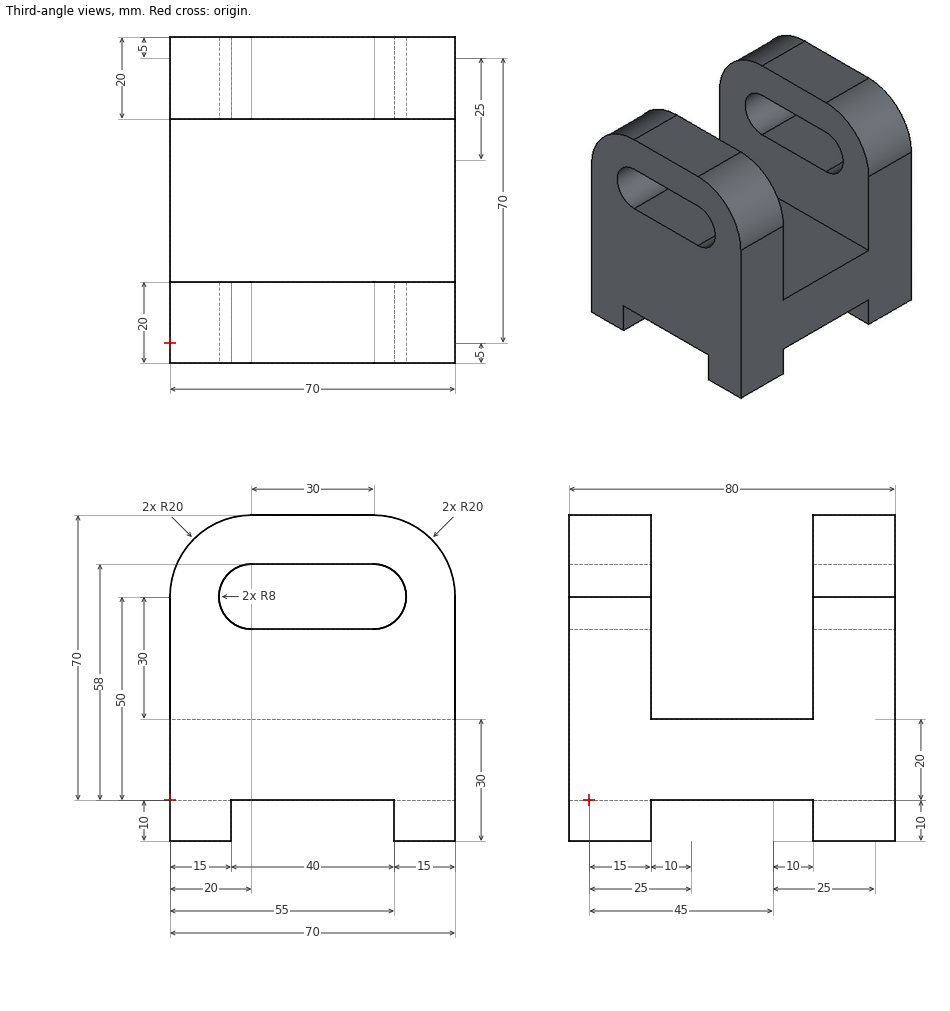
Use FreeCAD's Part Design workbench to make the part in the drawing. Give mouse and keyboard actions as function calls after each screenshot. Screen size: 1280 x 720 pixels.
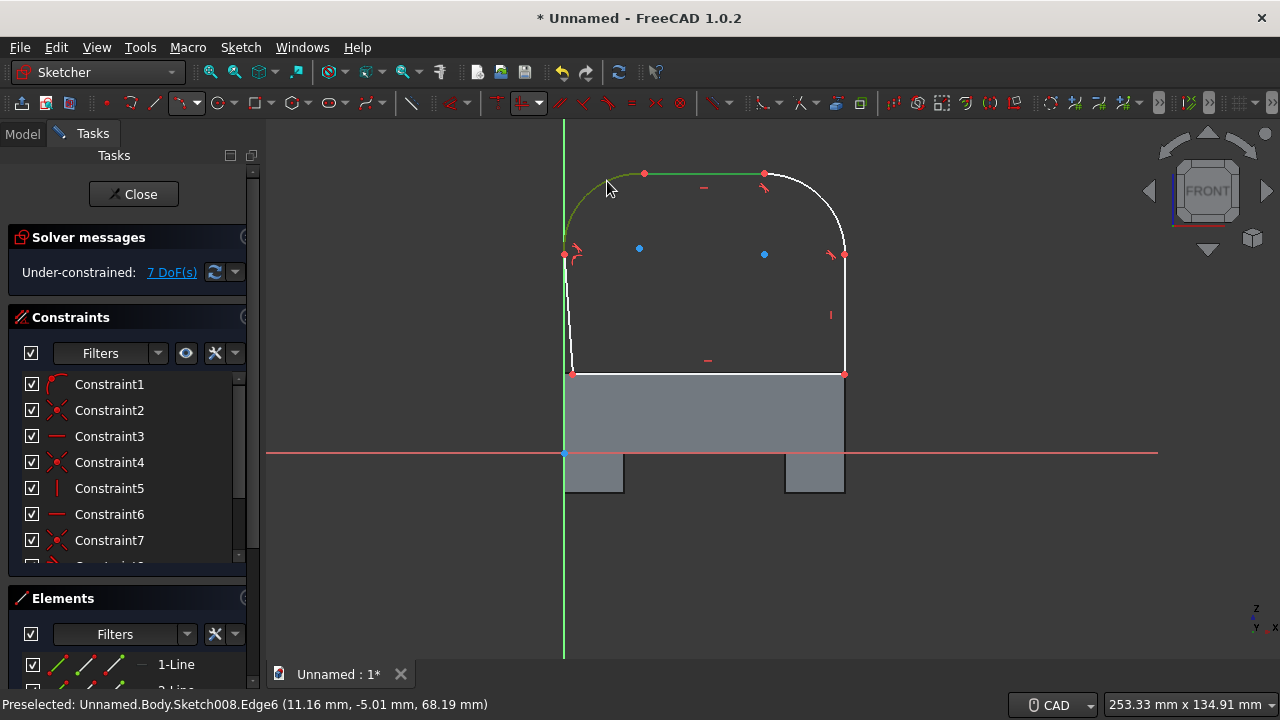
key(t)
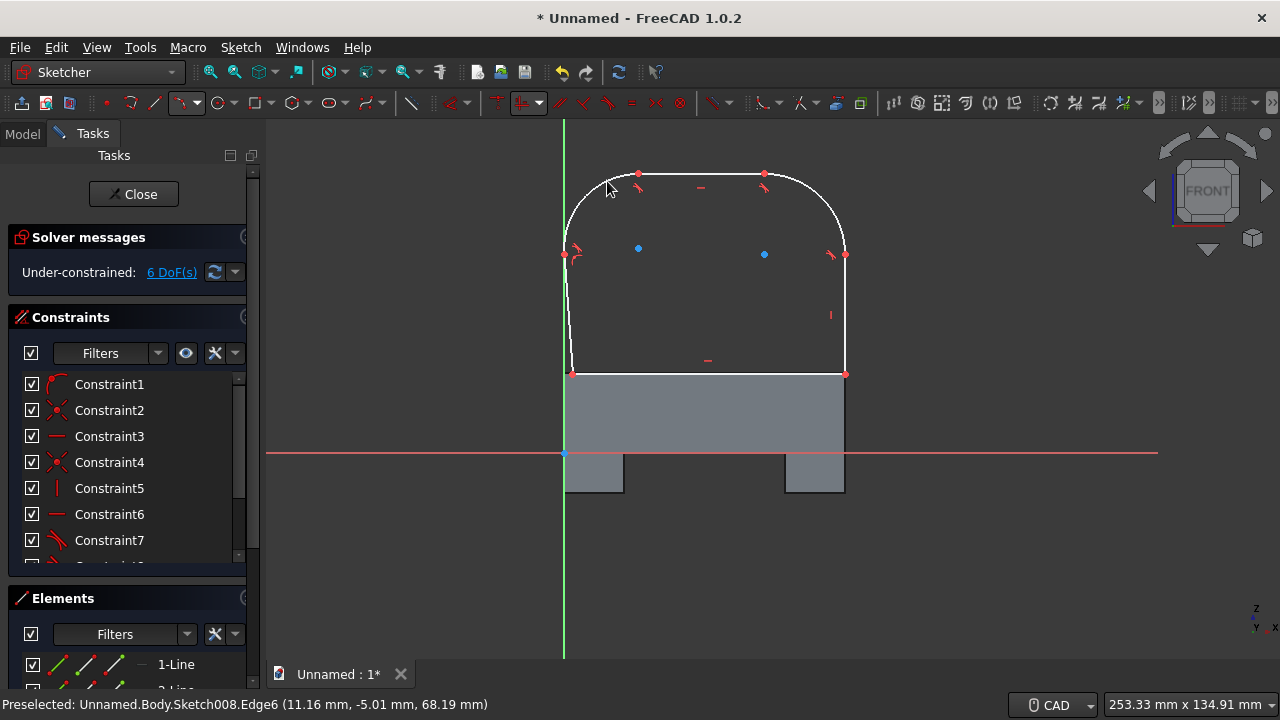
click(567, 290)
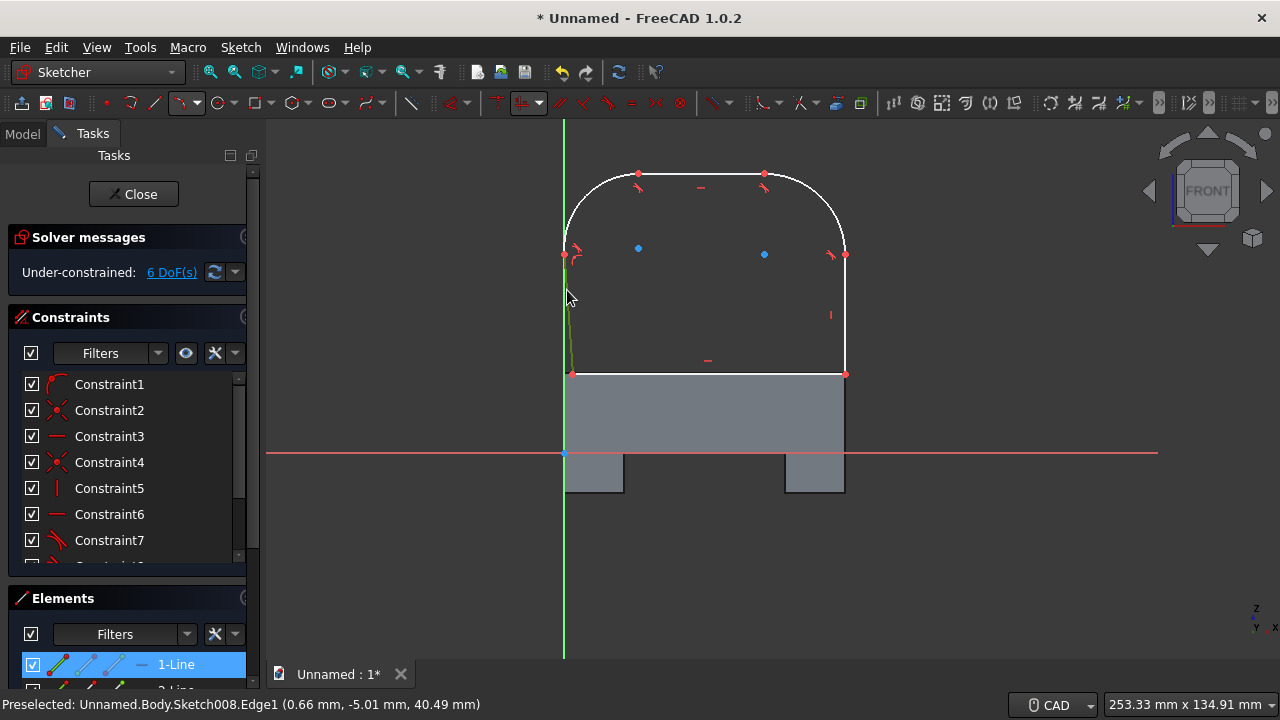
key(v)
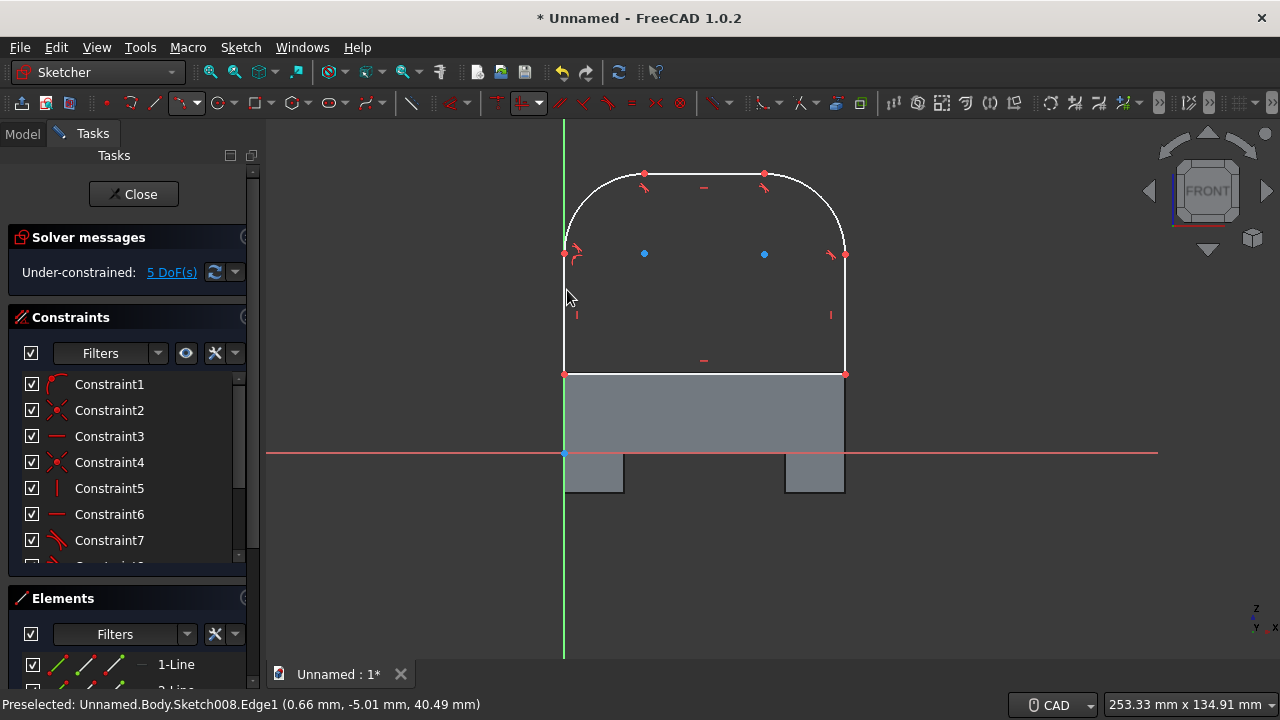
click(836, 218)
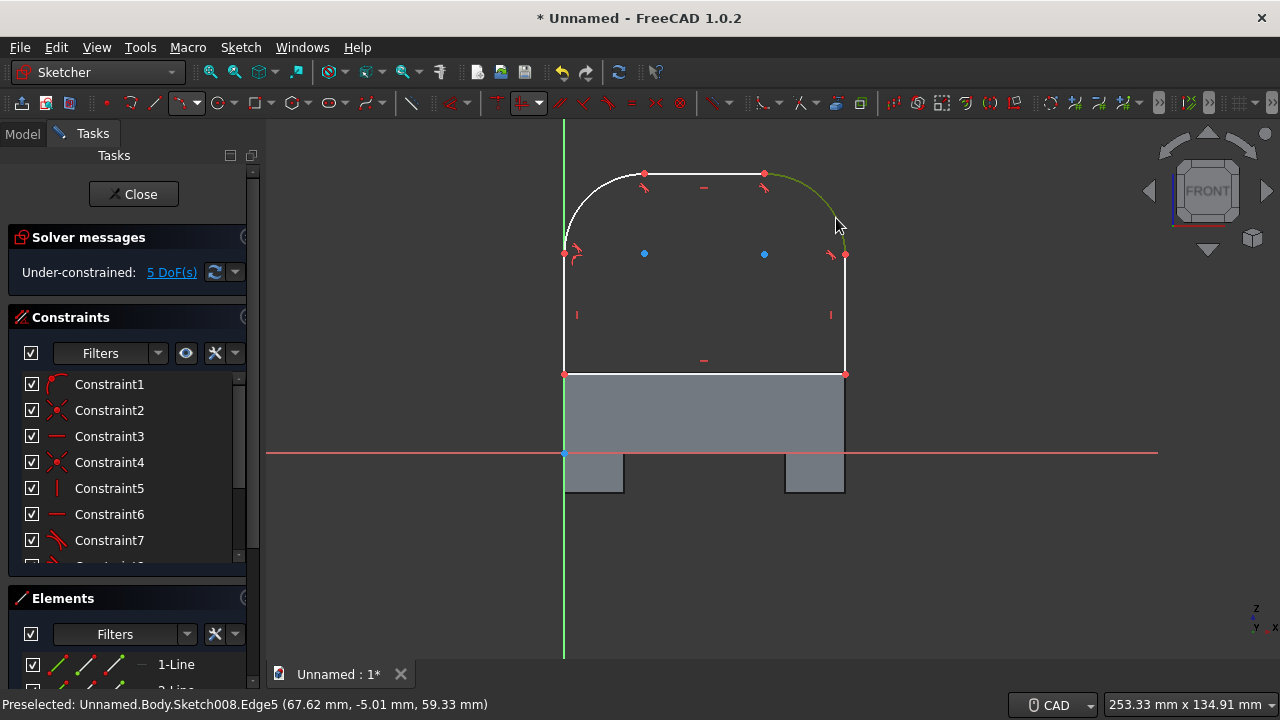
click(608, 183)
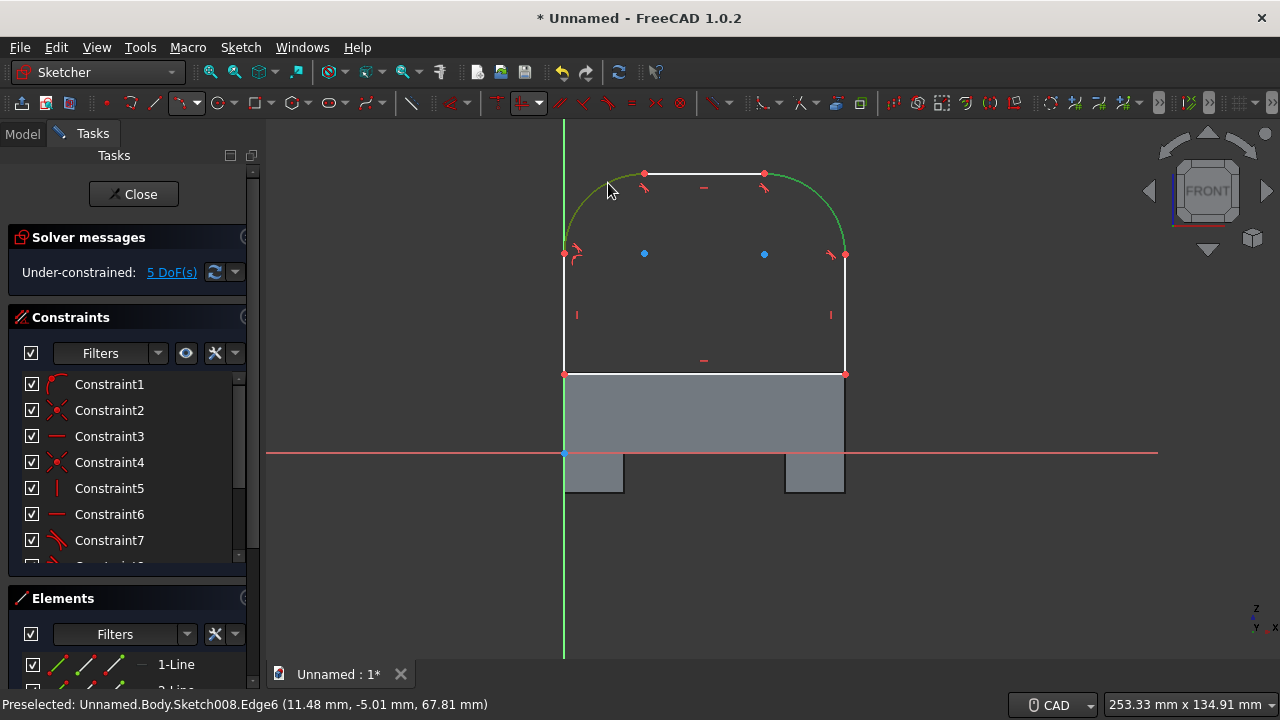
key(e)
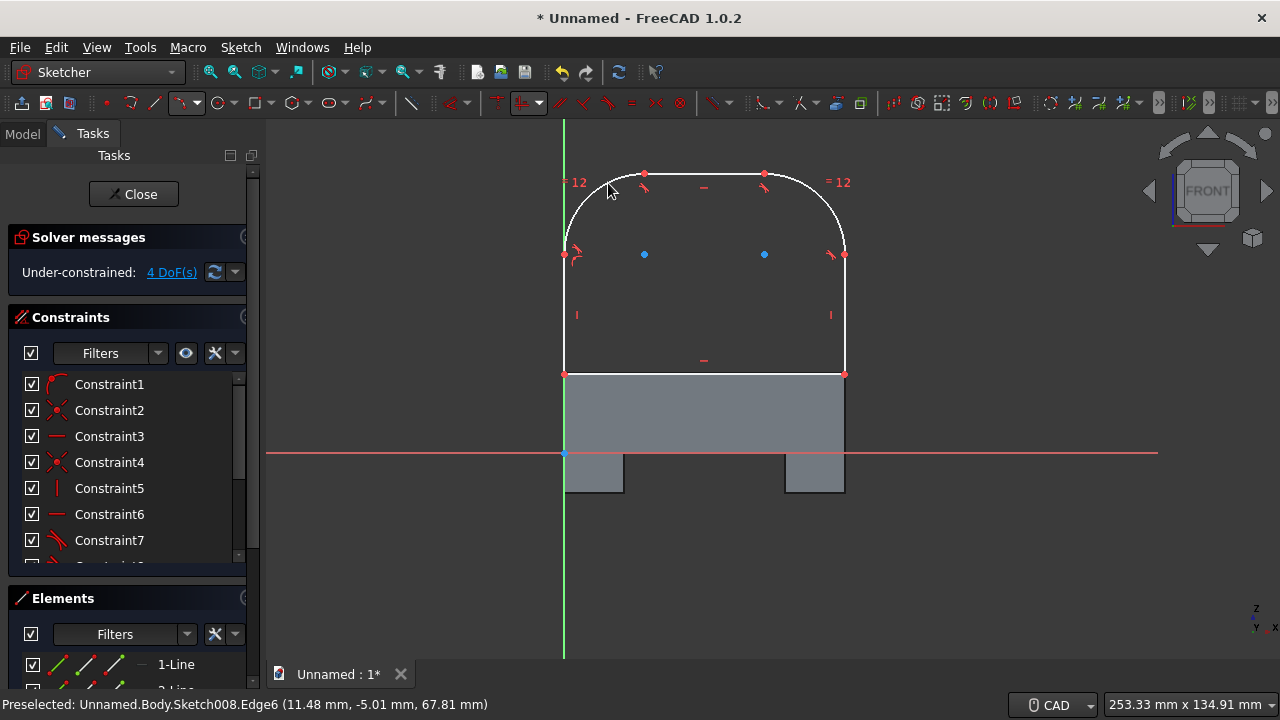
key(d)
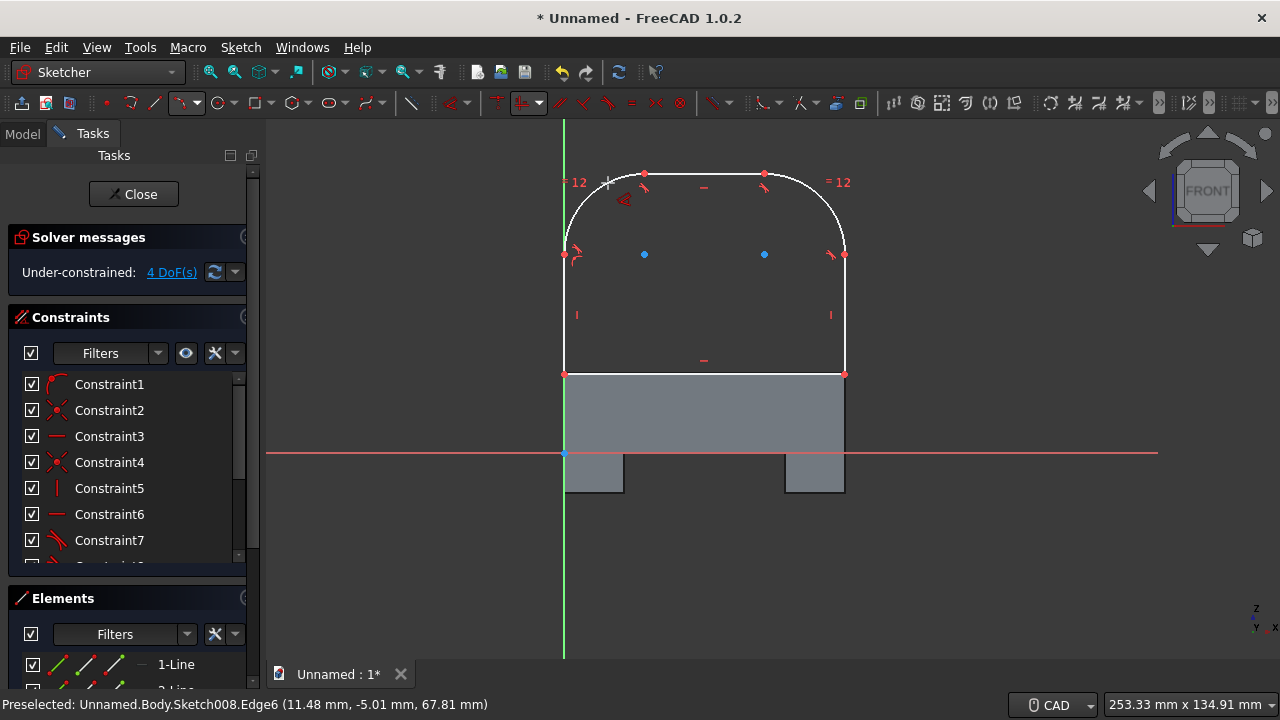
click(836, 218)
click(865, 203)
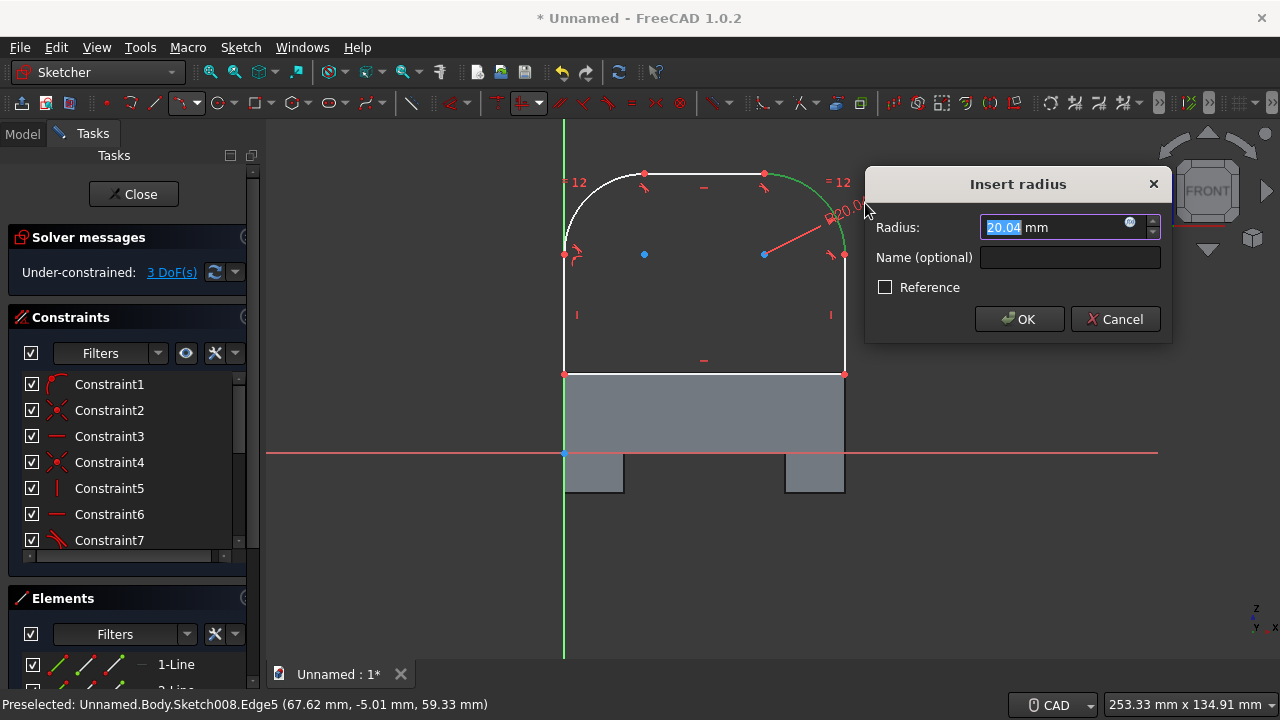
text(20)
key(Return)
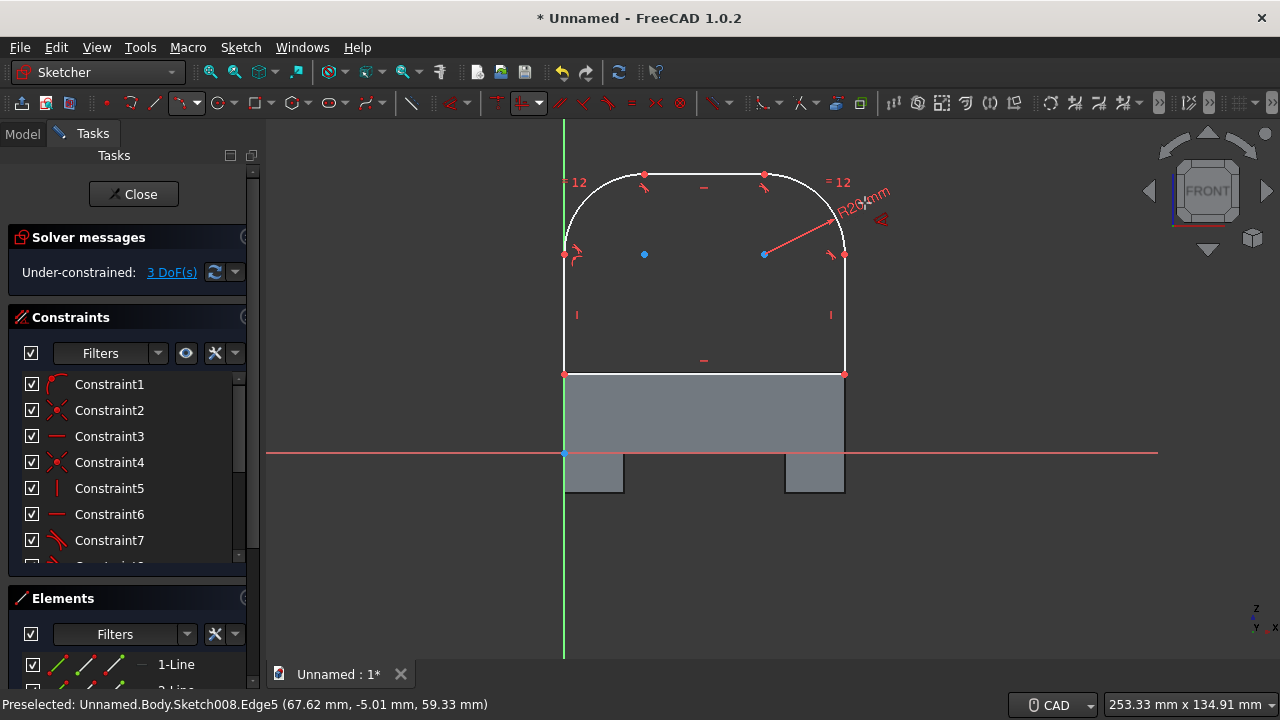
click(564, 290)
click(530, 314)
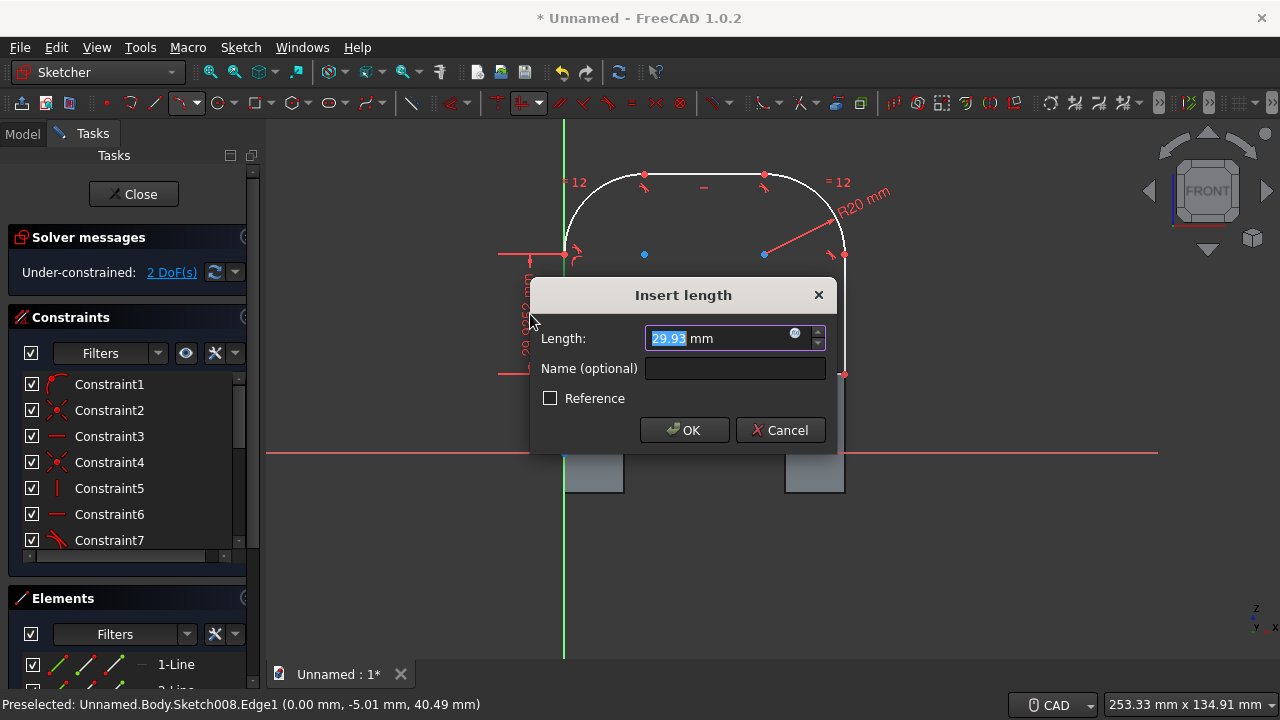
text(30)
key(Return)